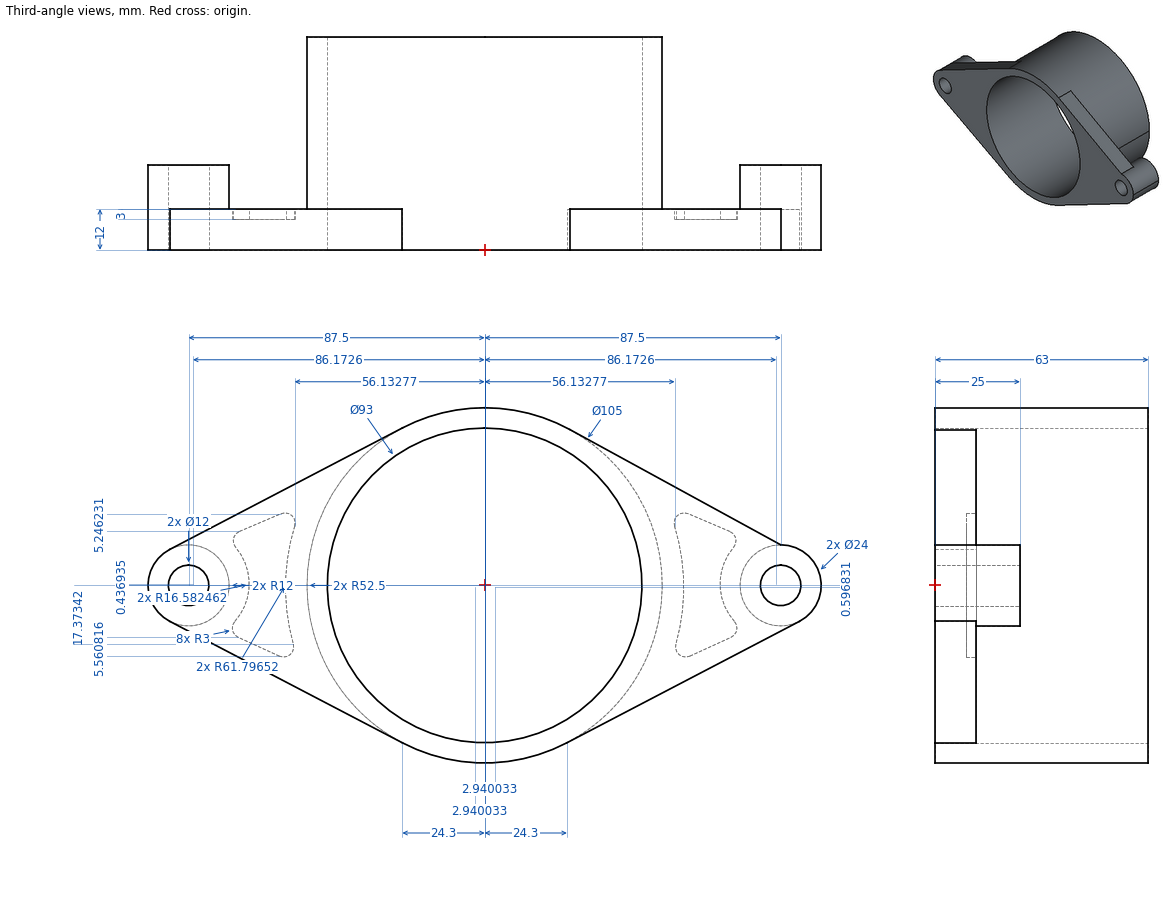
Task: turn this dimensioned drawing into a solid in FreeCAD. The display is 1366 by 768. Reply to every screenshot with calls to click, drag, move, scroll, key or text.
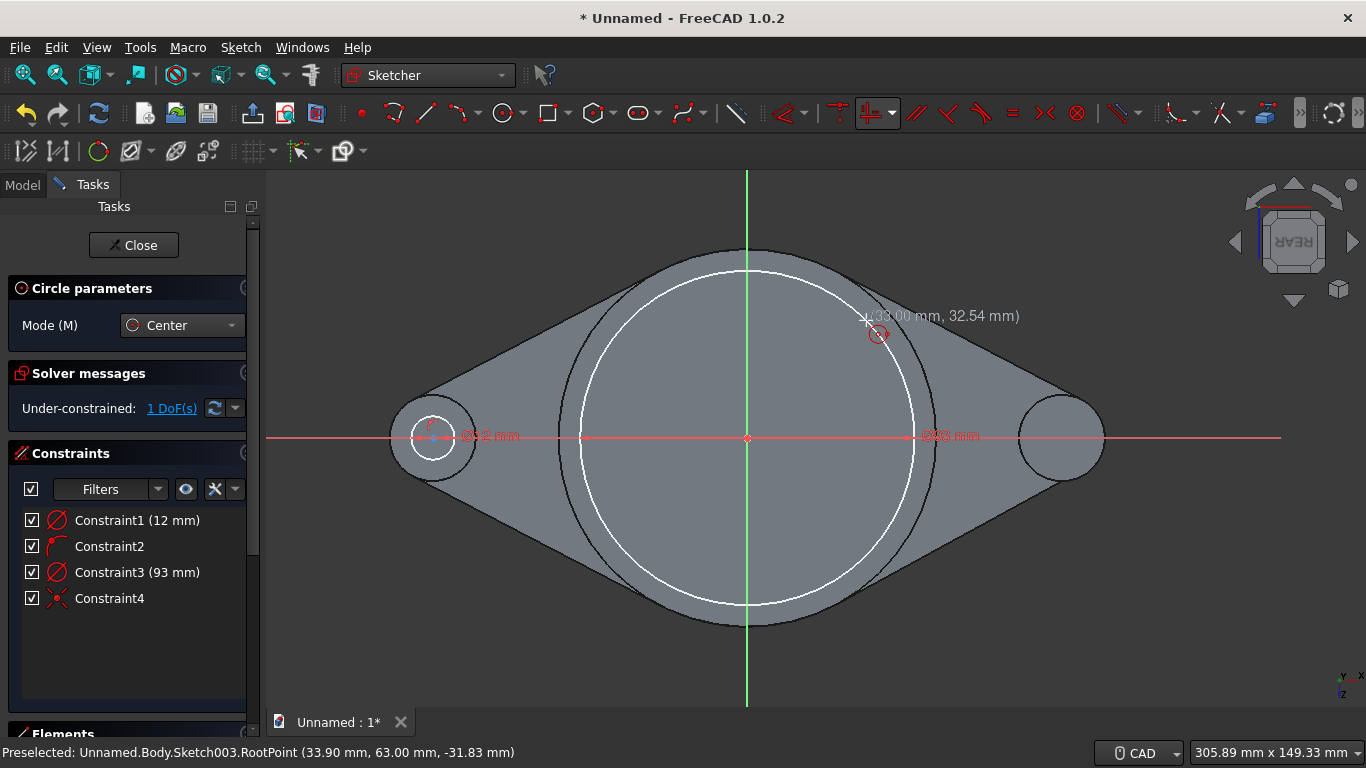
click(1062, 438)
move(1077, 423)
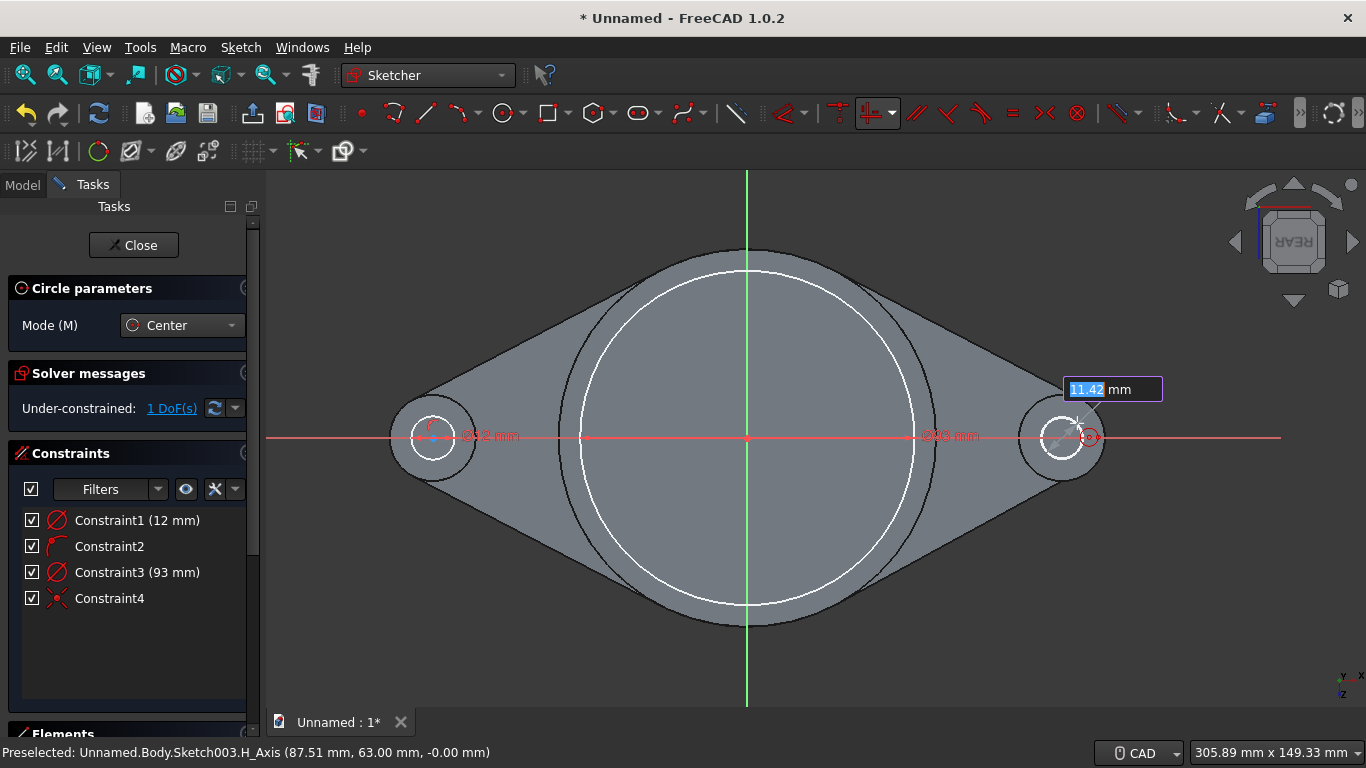
text(12)
key(Return)
key(Escape)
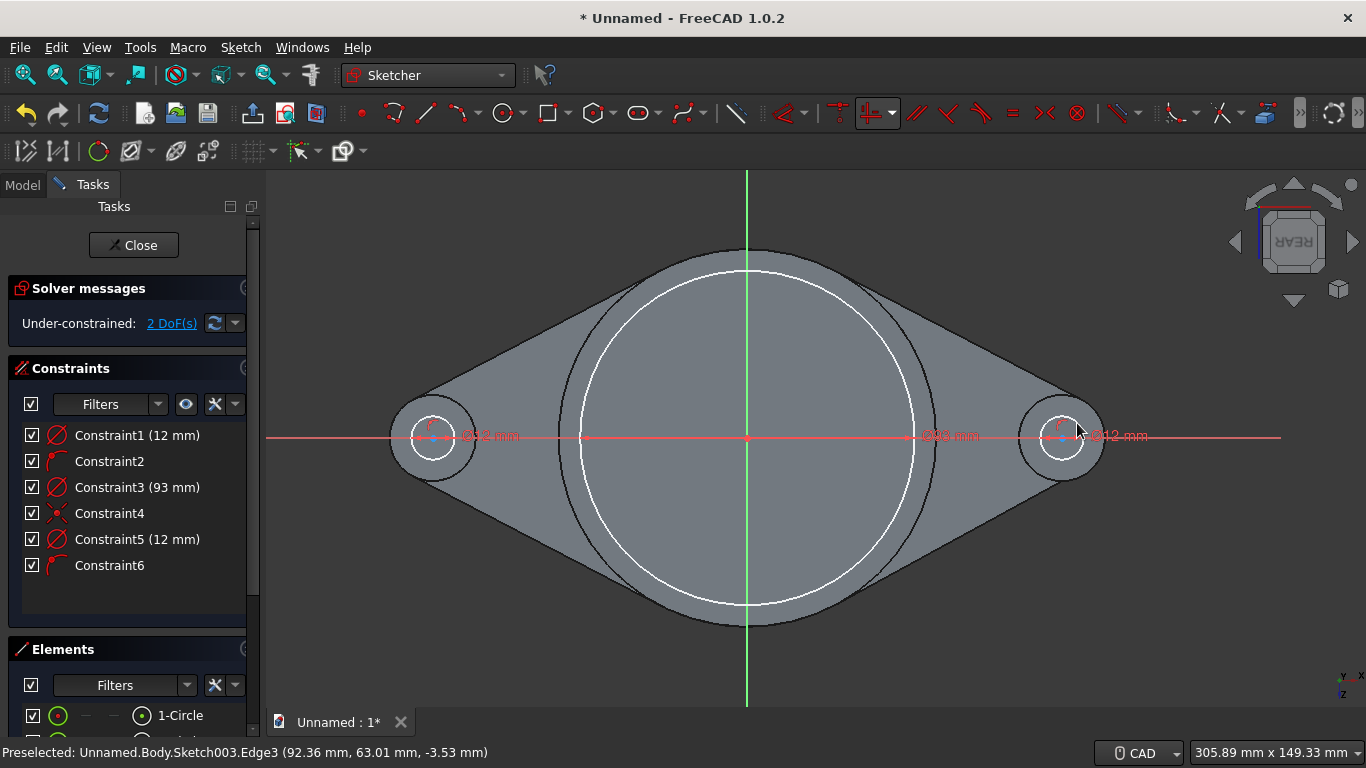
key(d)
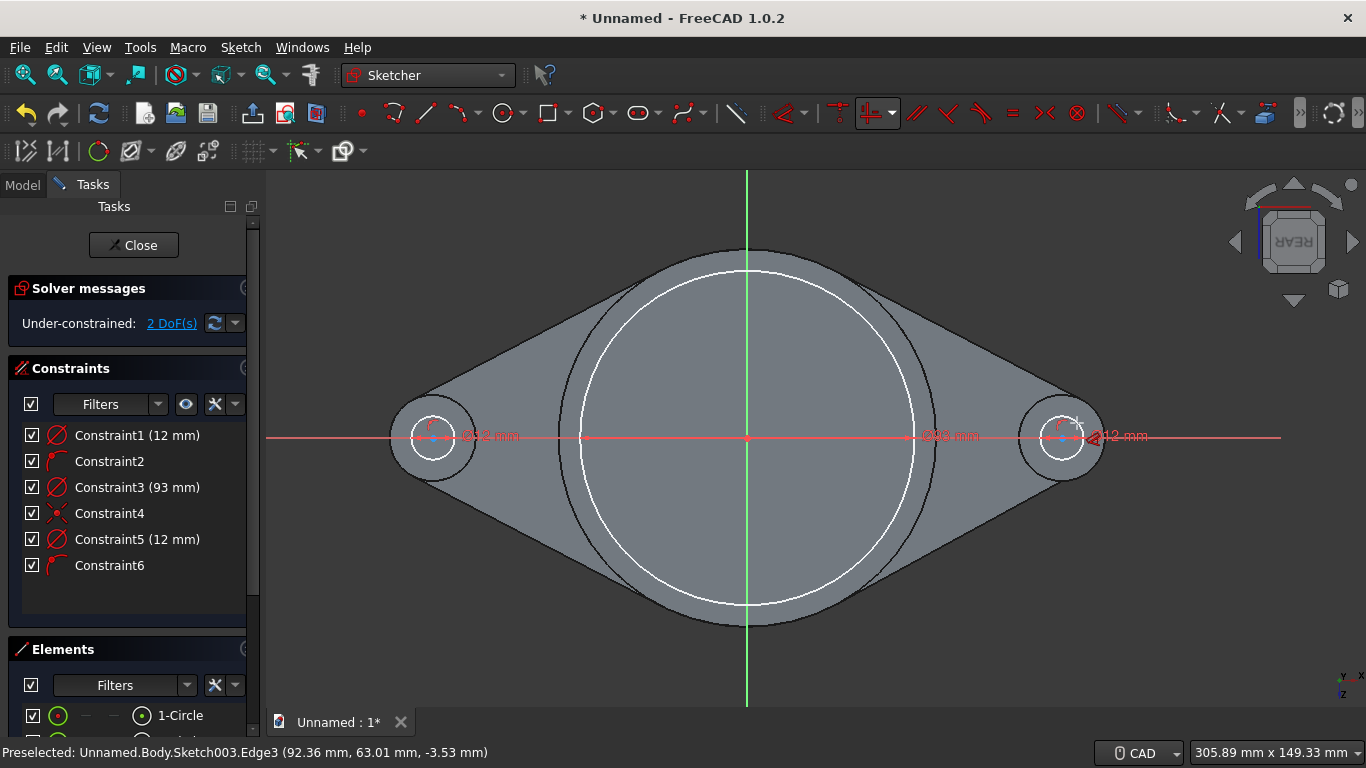
click(433, 438)
click(518, 472)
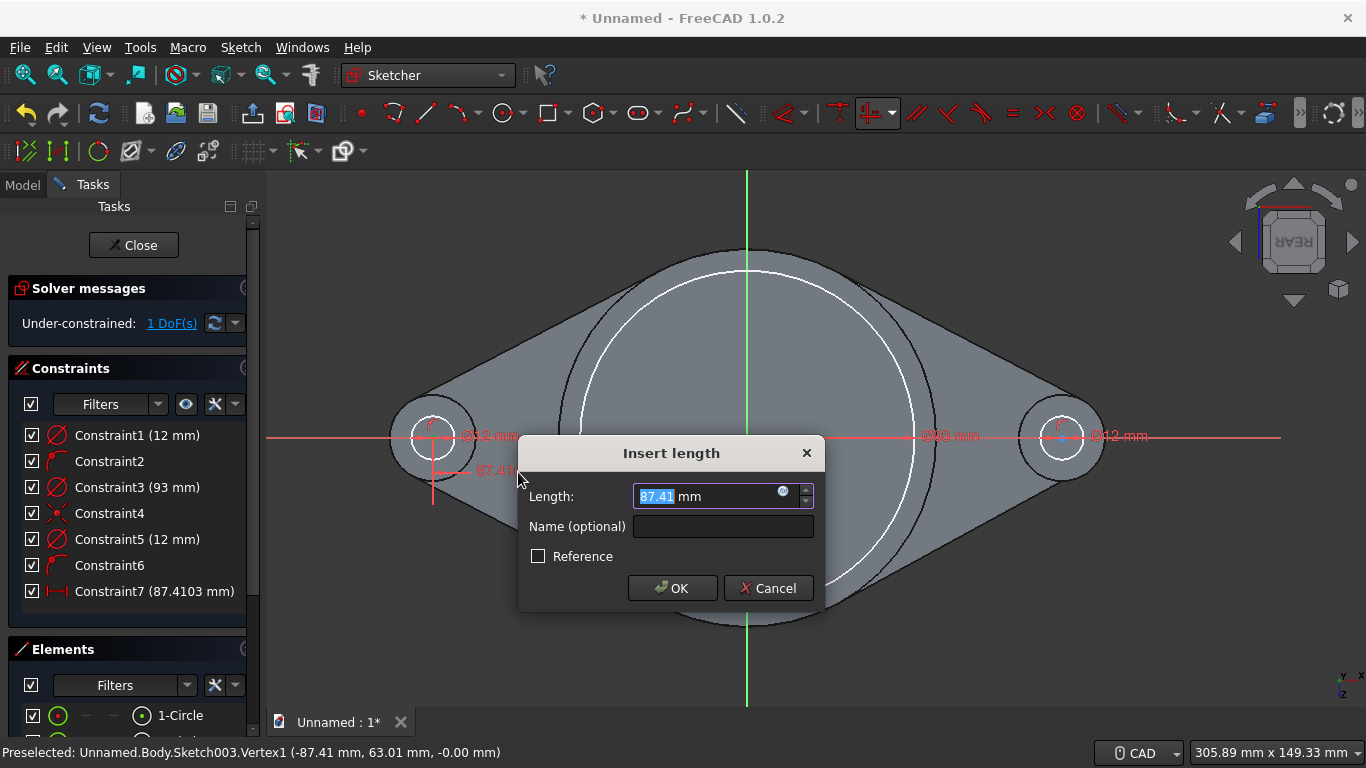
text(87.5)
key(Return)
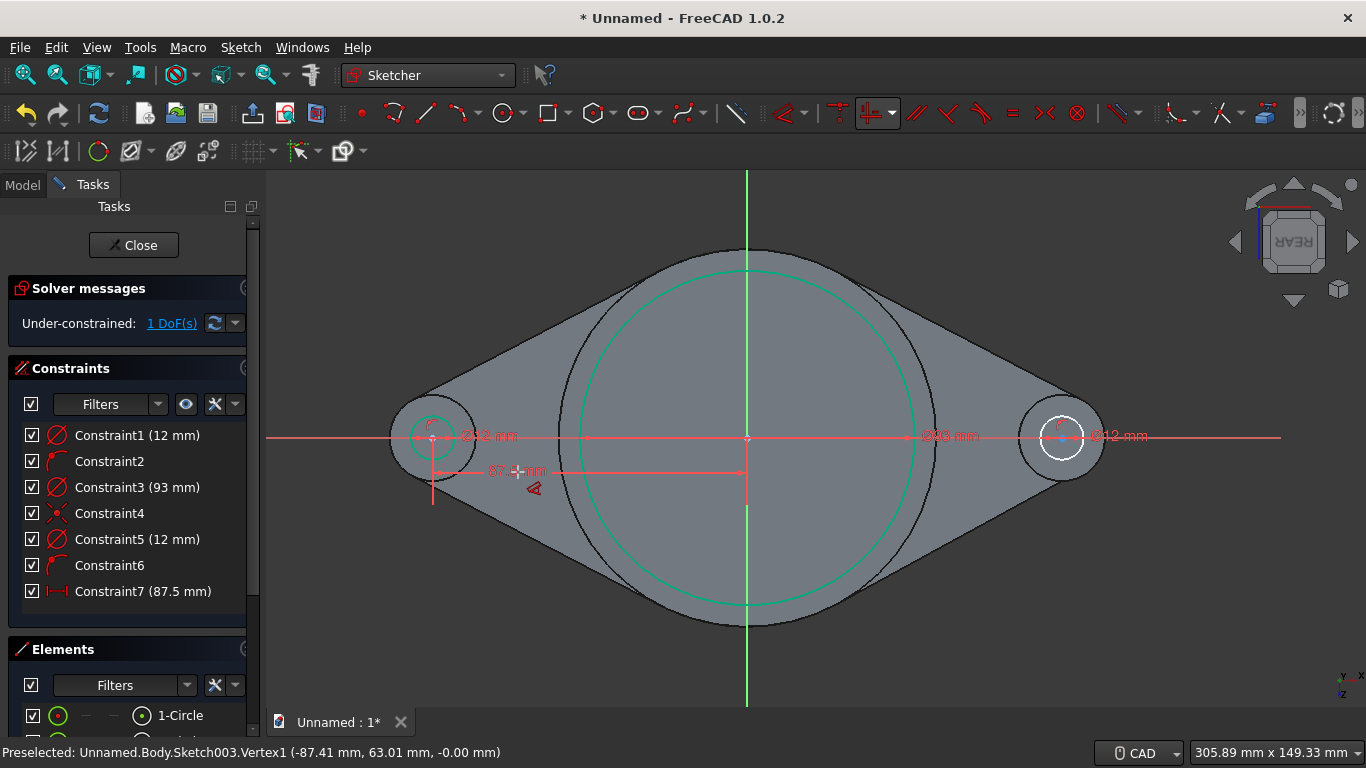
click(1062, 438)
click(832, 472)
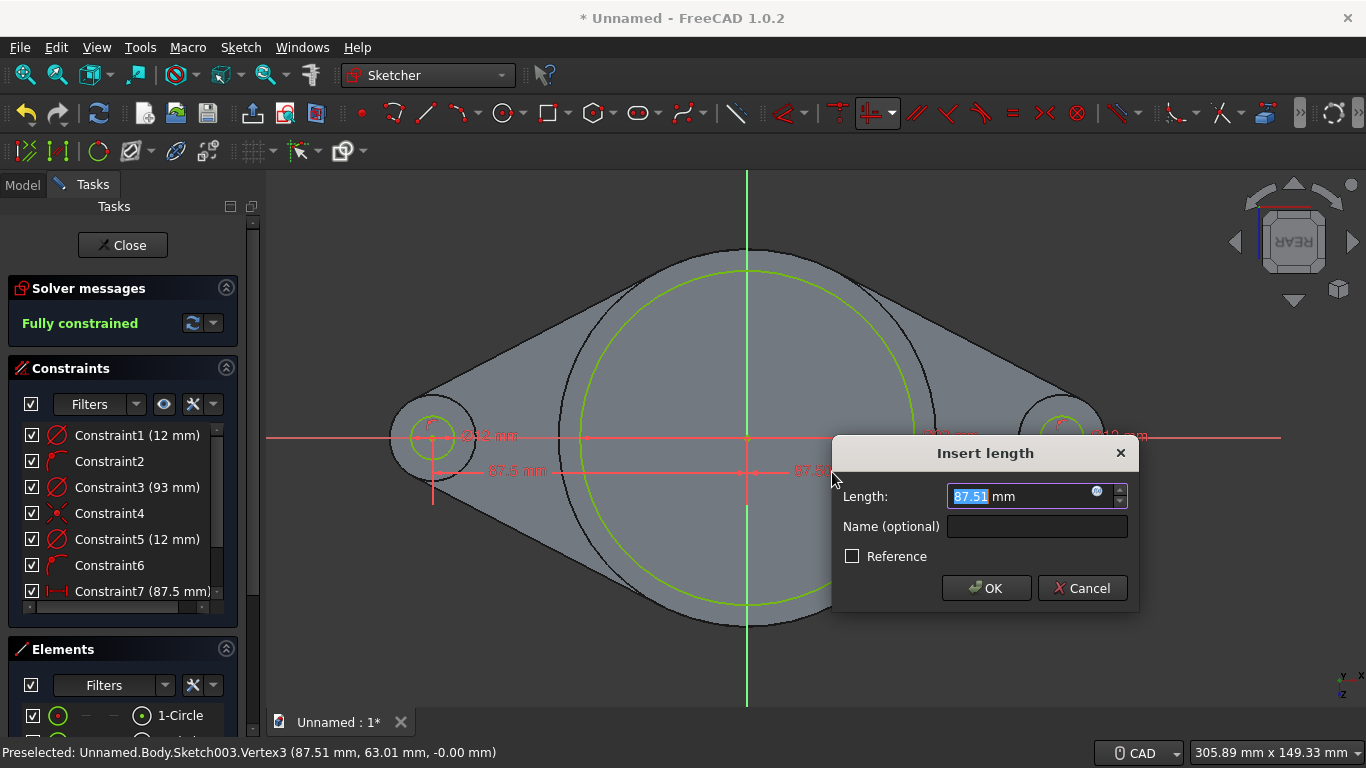
text(87.5)
key(Return)
key(Escape)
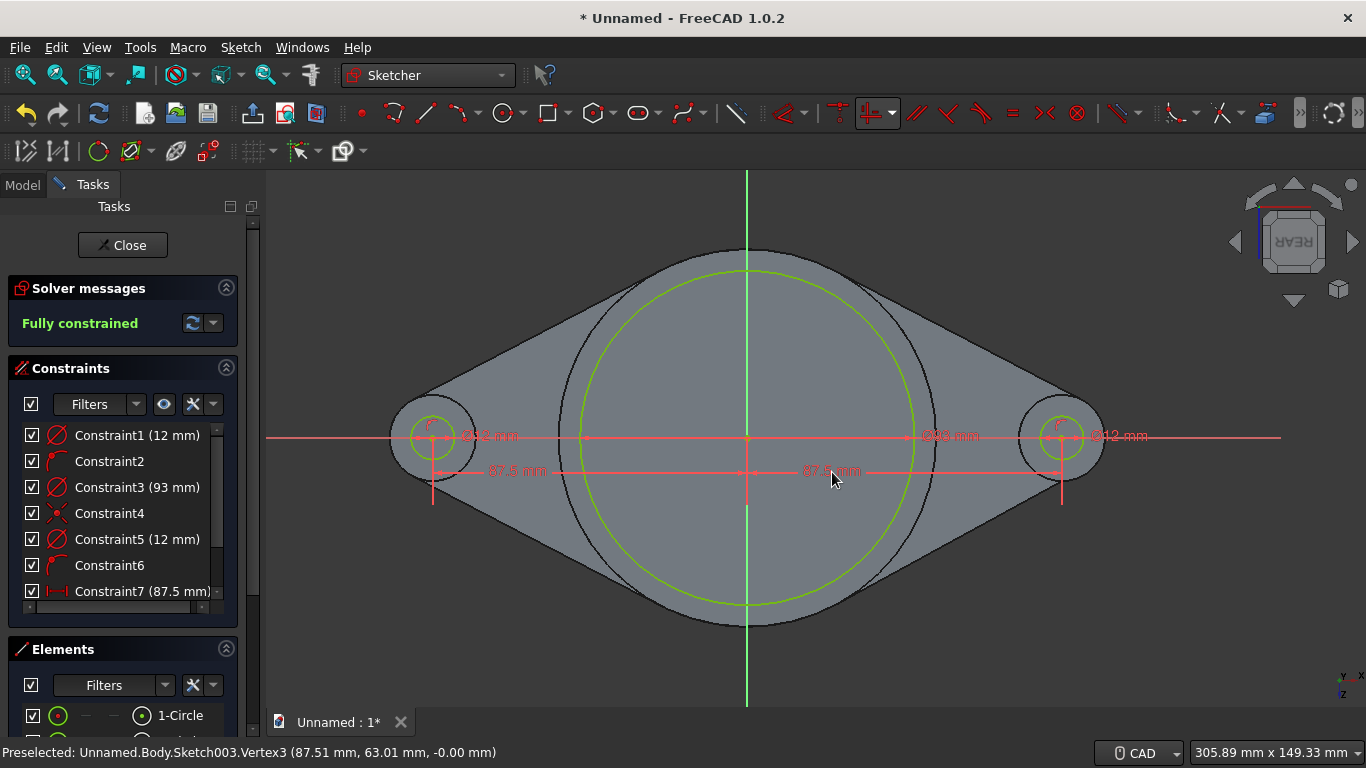
click(123, 245)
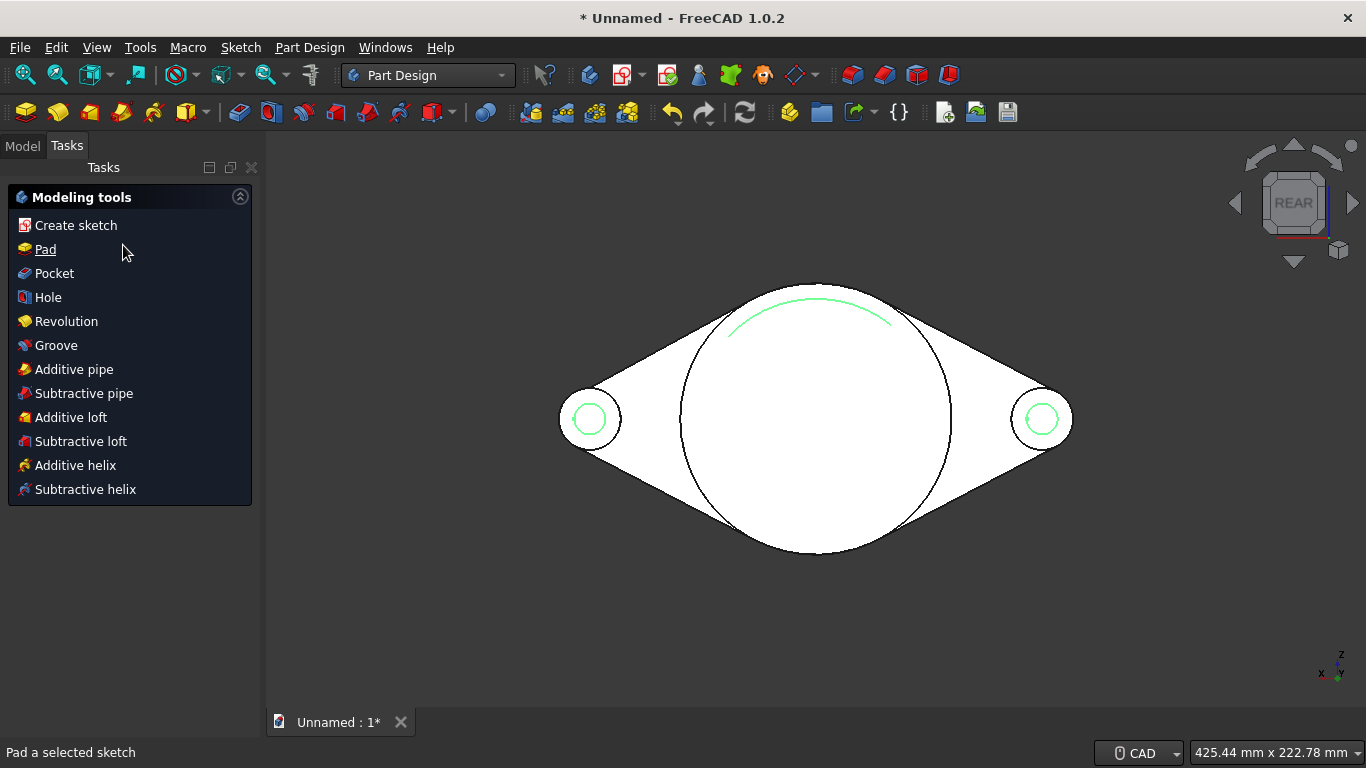
click(240, 112)